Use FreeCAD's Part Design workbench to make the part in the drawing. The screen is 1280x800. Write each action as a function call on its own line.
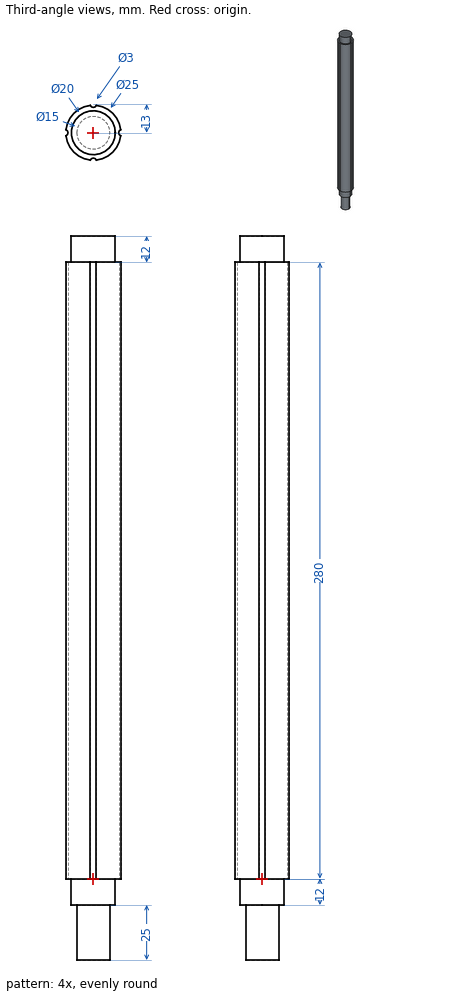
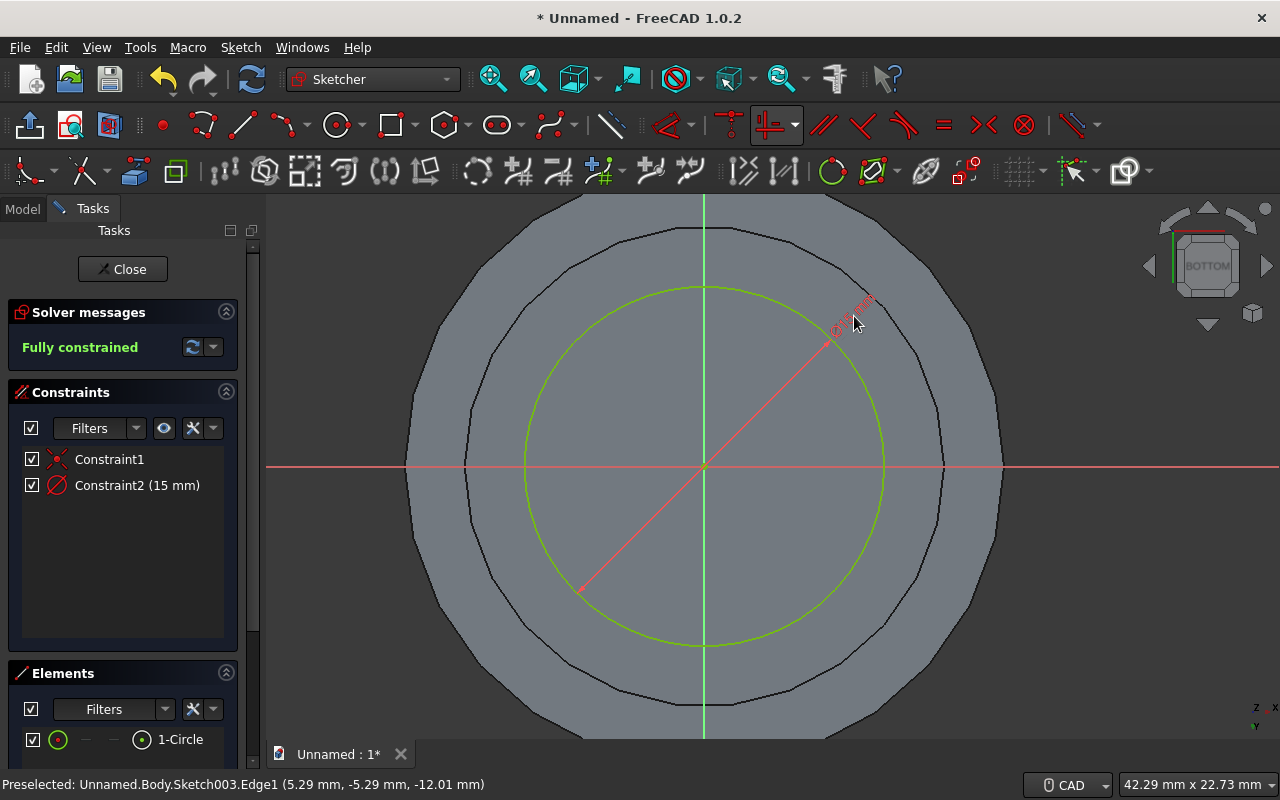
click(123, 269)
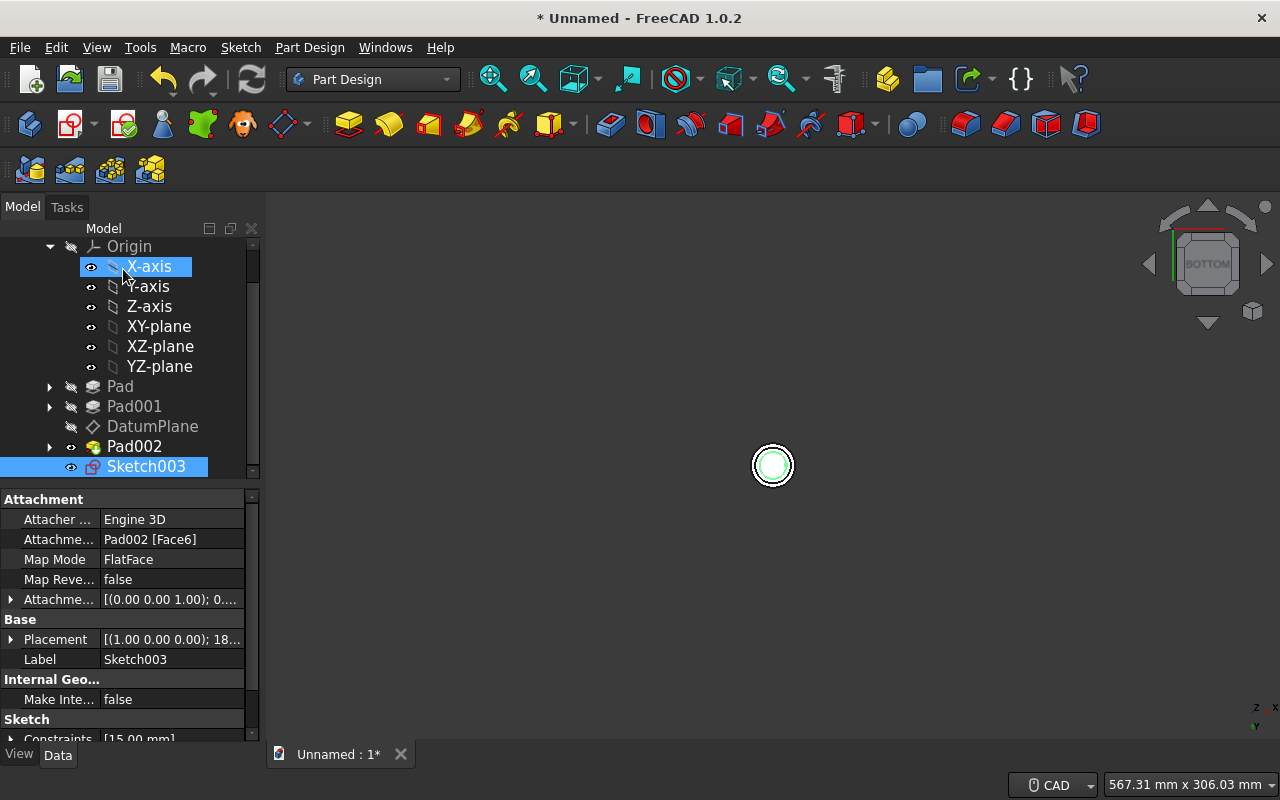
click(350, 124)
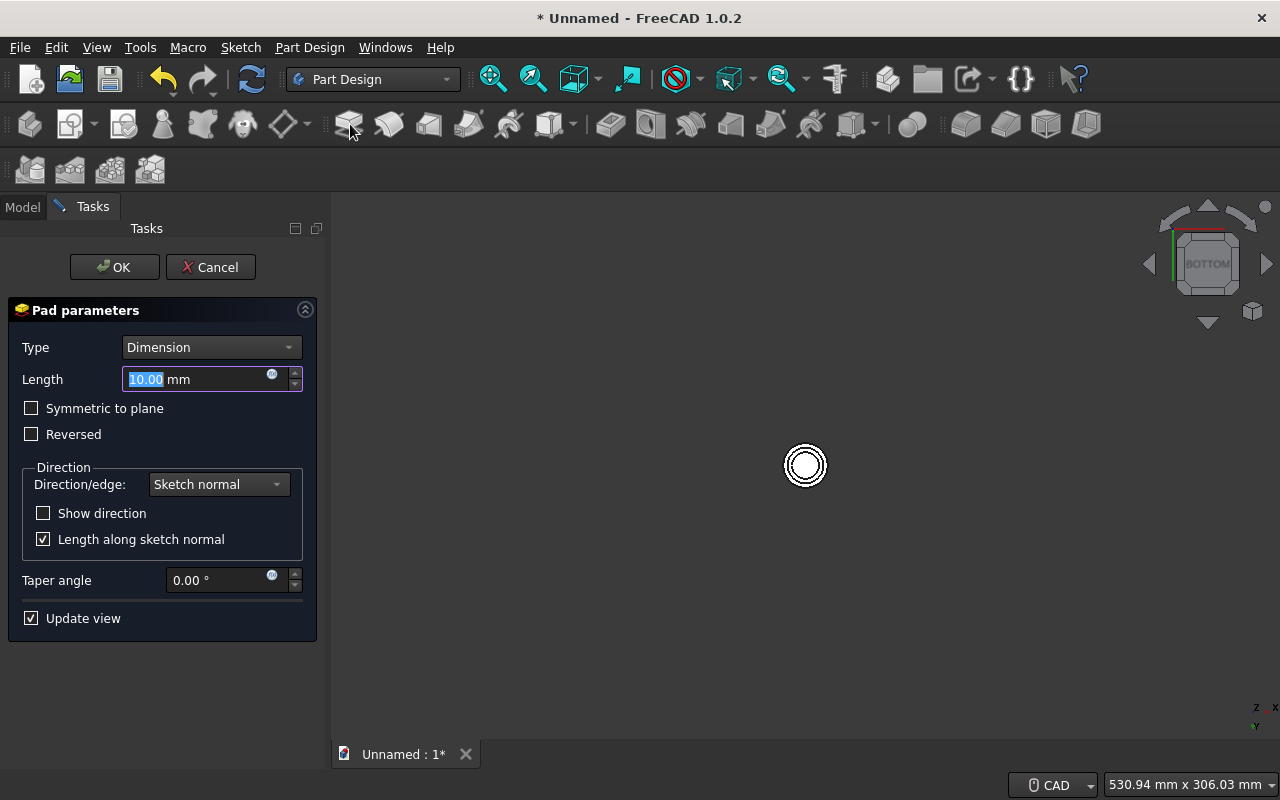
text(25)
key(Tab)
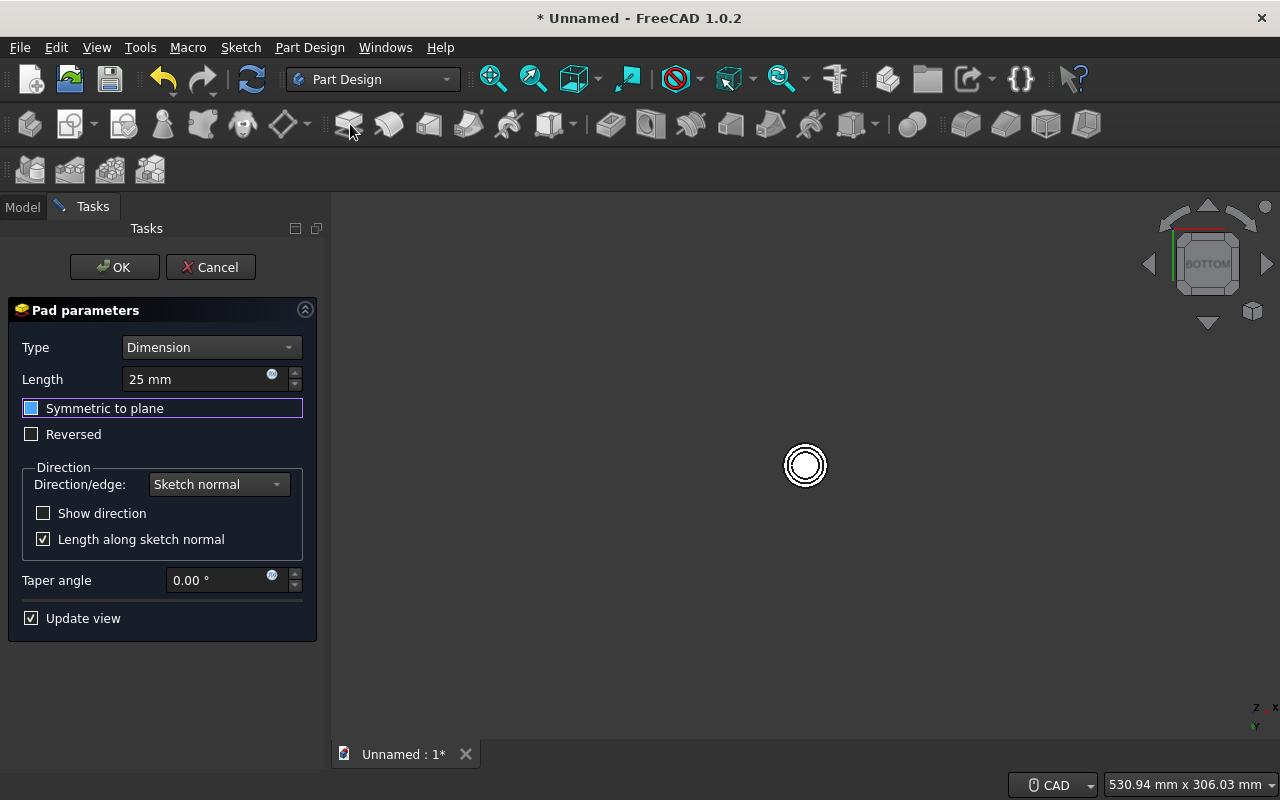
click(115, 267)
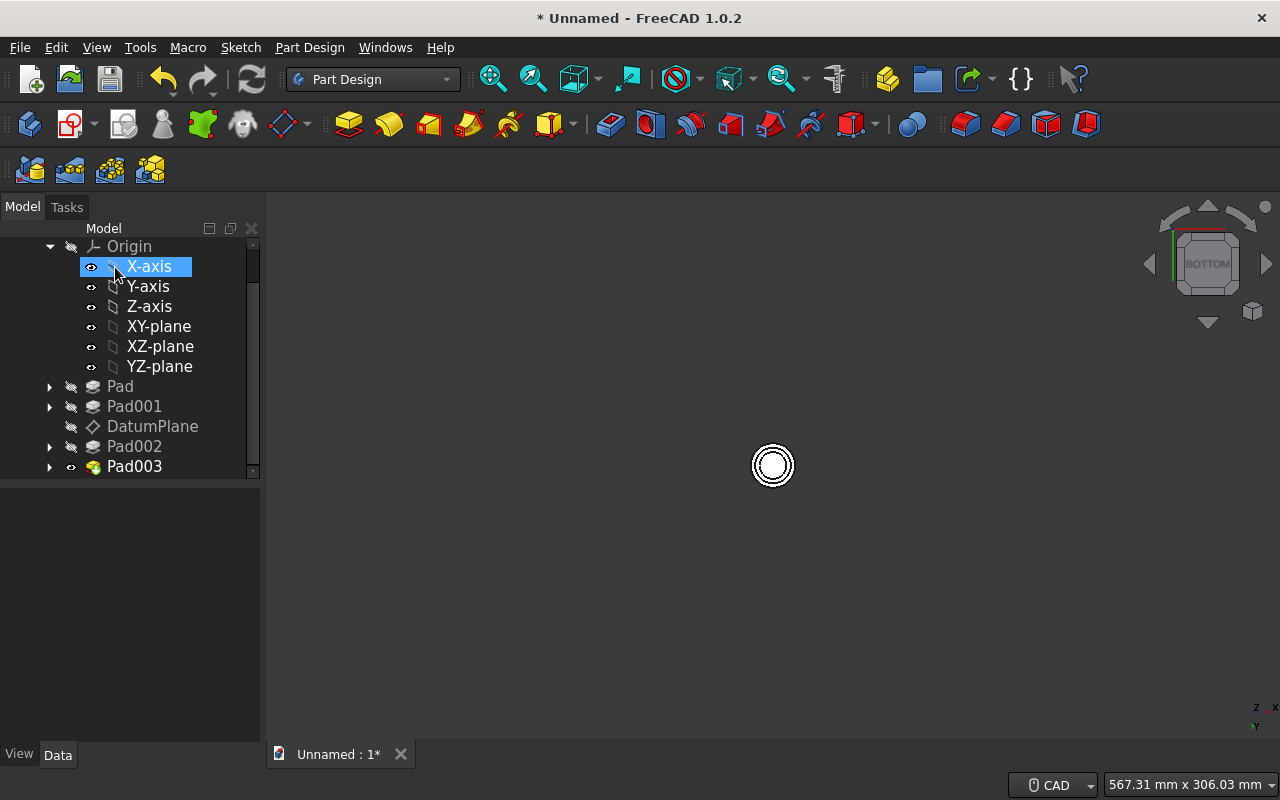
key(v)
key(f)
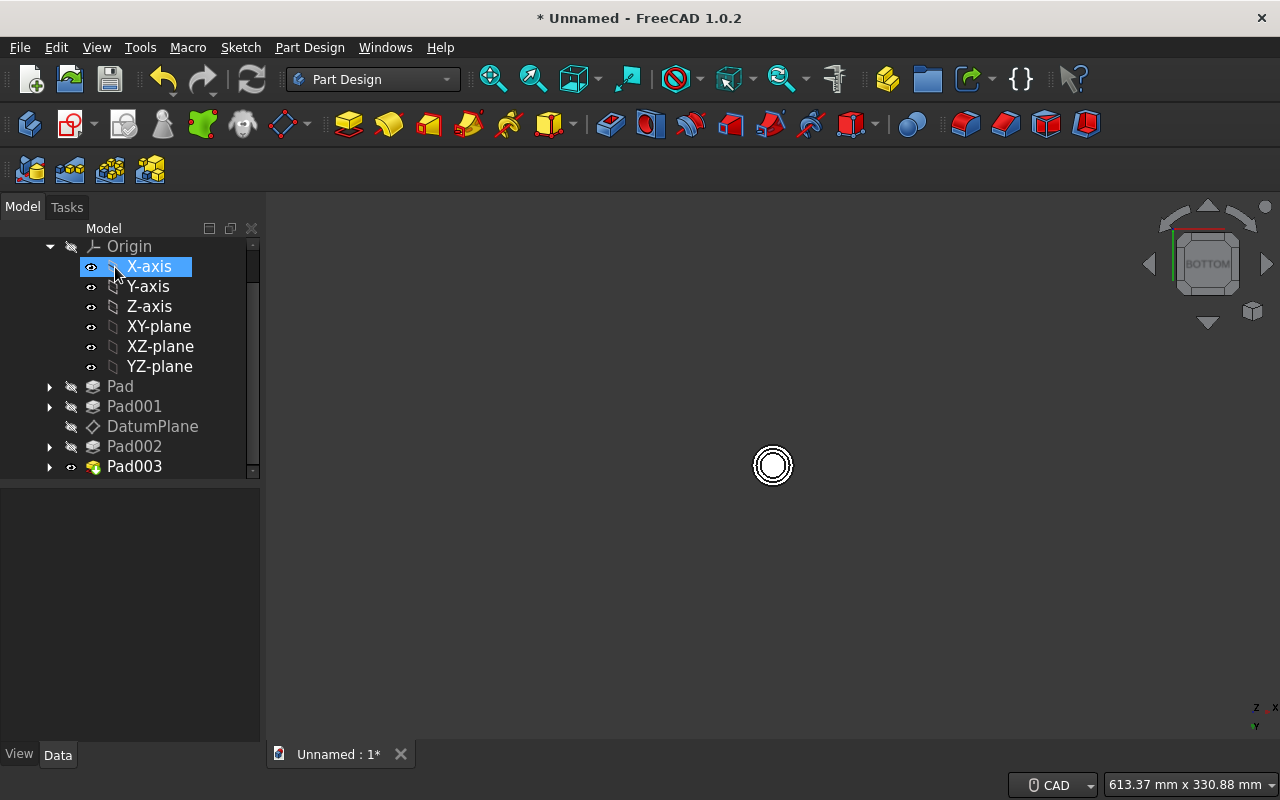
scroll(755, 459, up, 9)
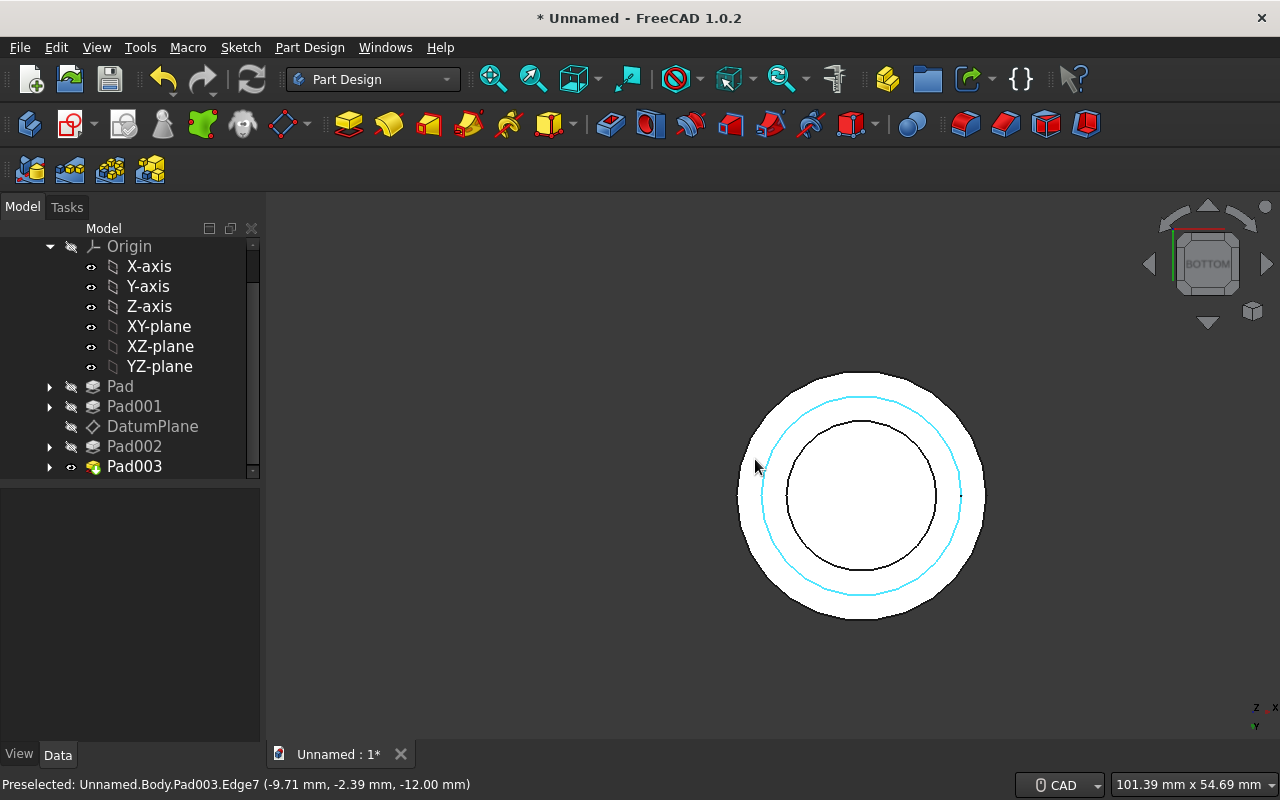
click(754, 459)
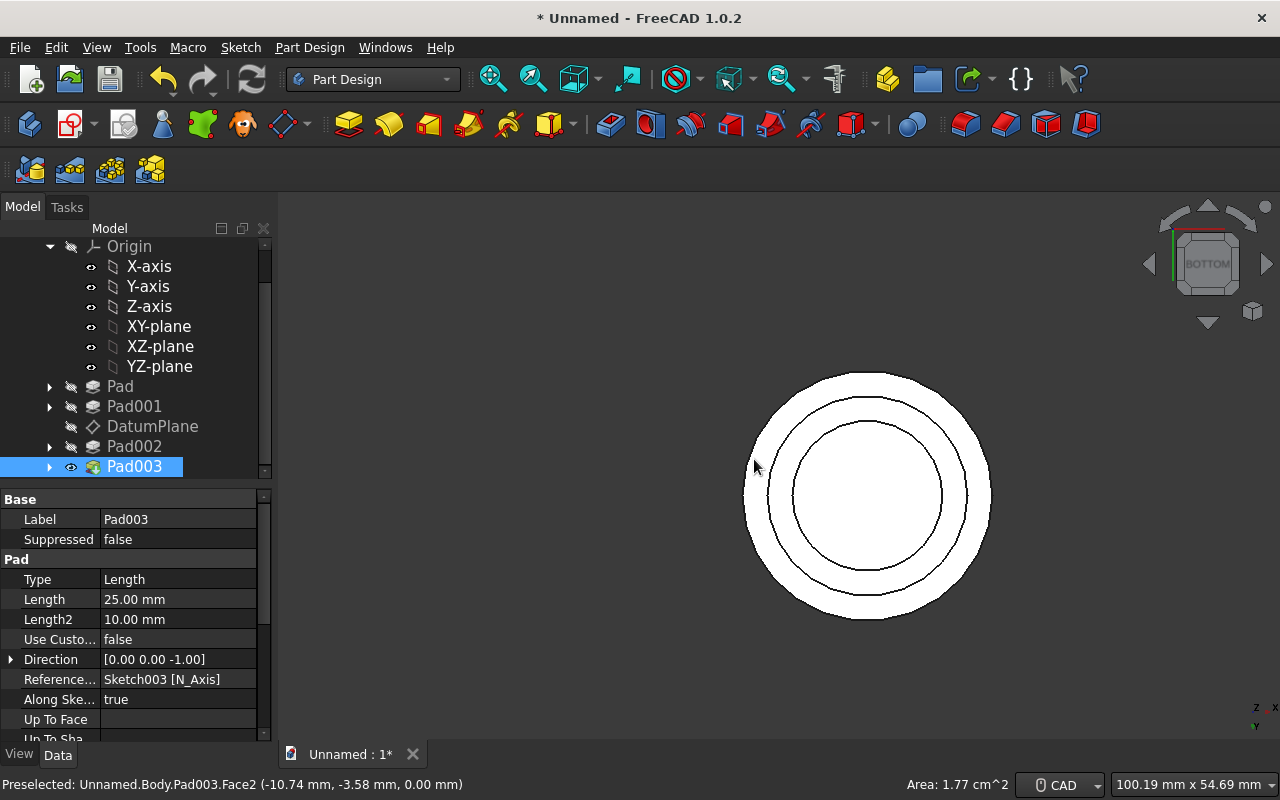
click(70, 124)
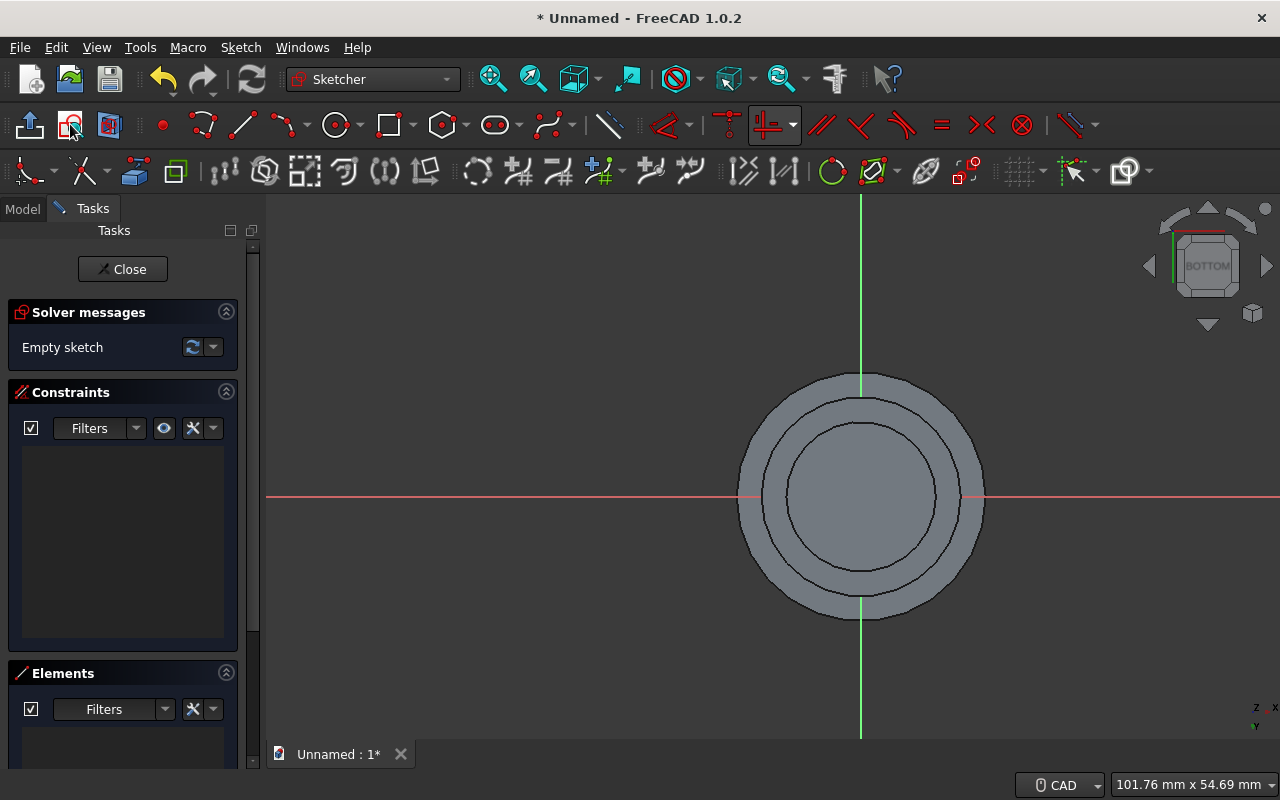
key(q)
key(s)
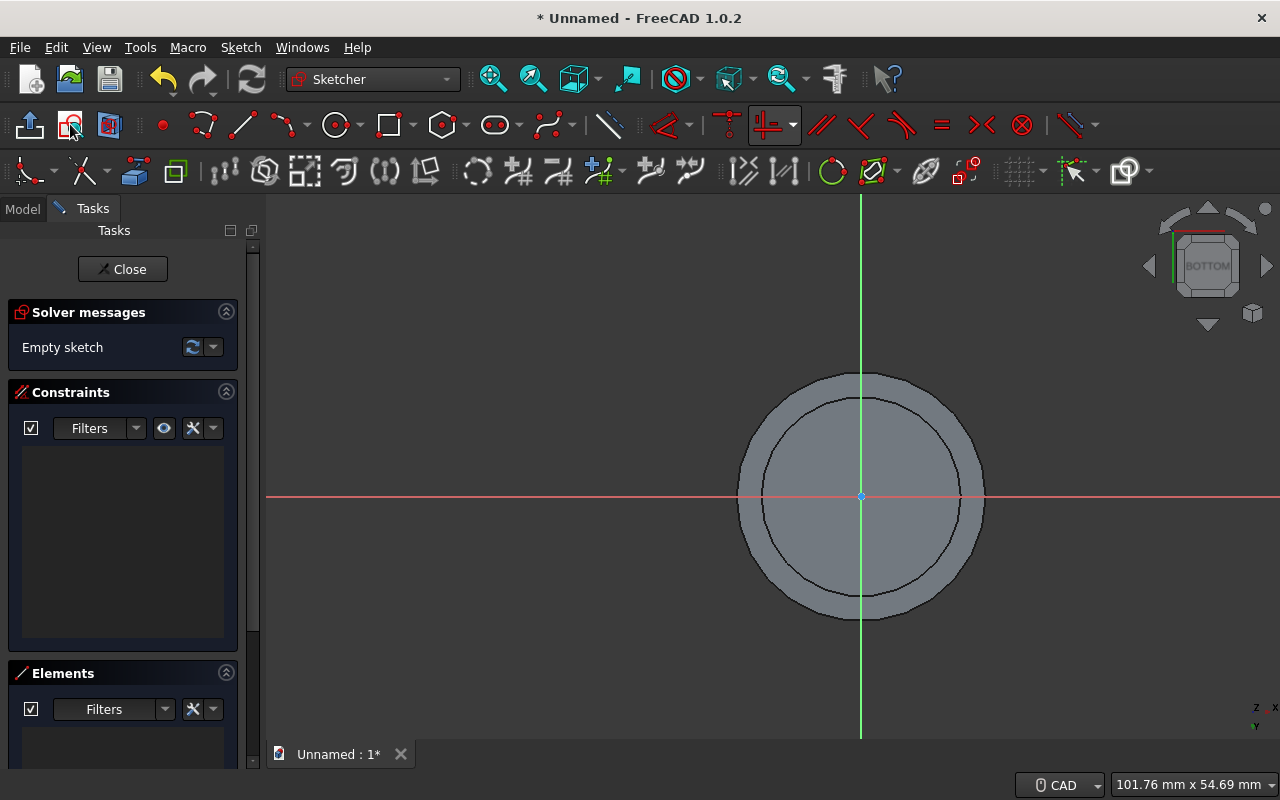
scroll(877, 642, up, 12)